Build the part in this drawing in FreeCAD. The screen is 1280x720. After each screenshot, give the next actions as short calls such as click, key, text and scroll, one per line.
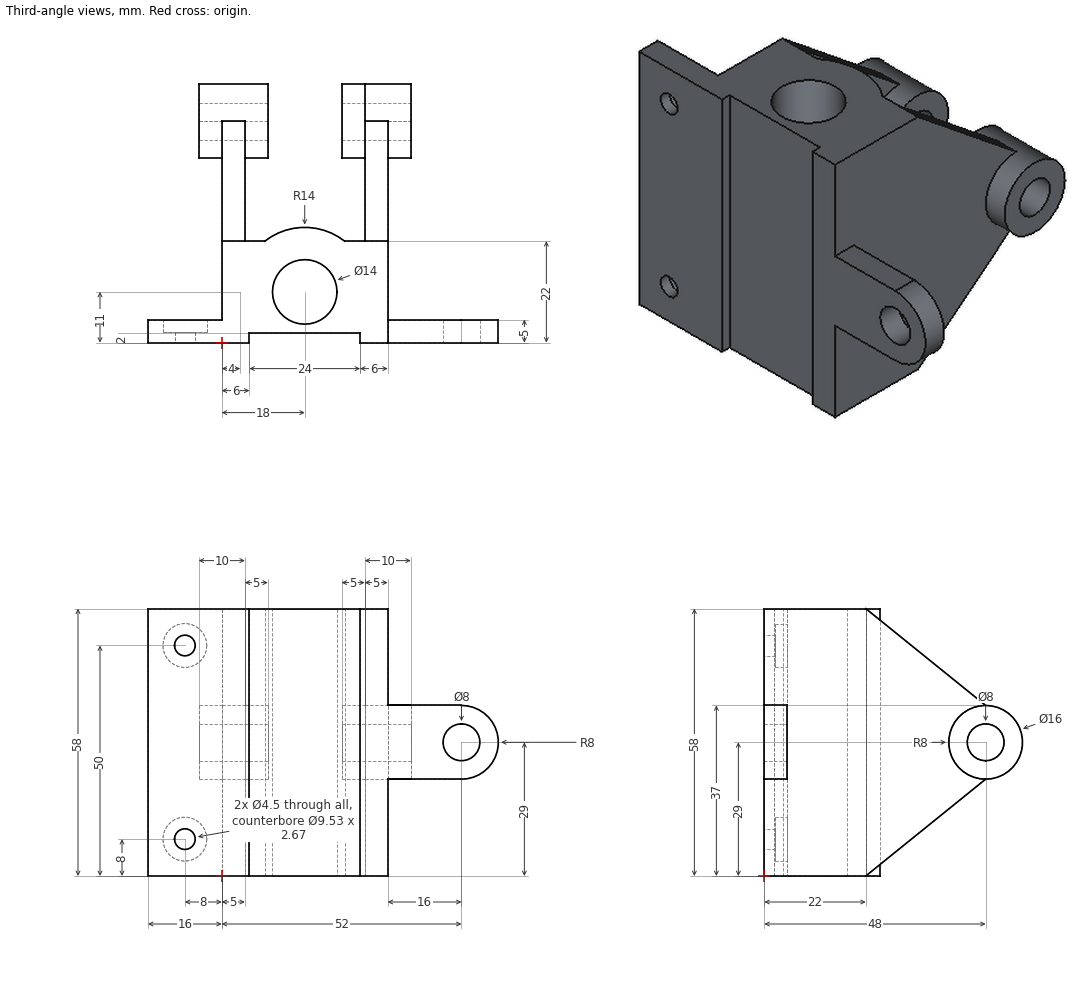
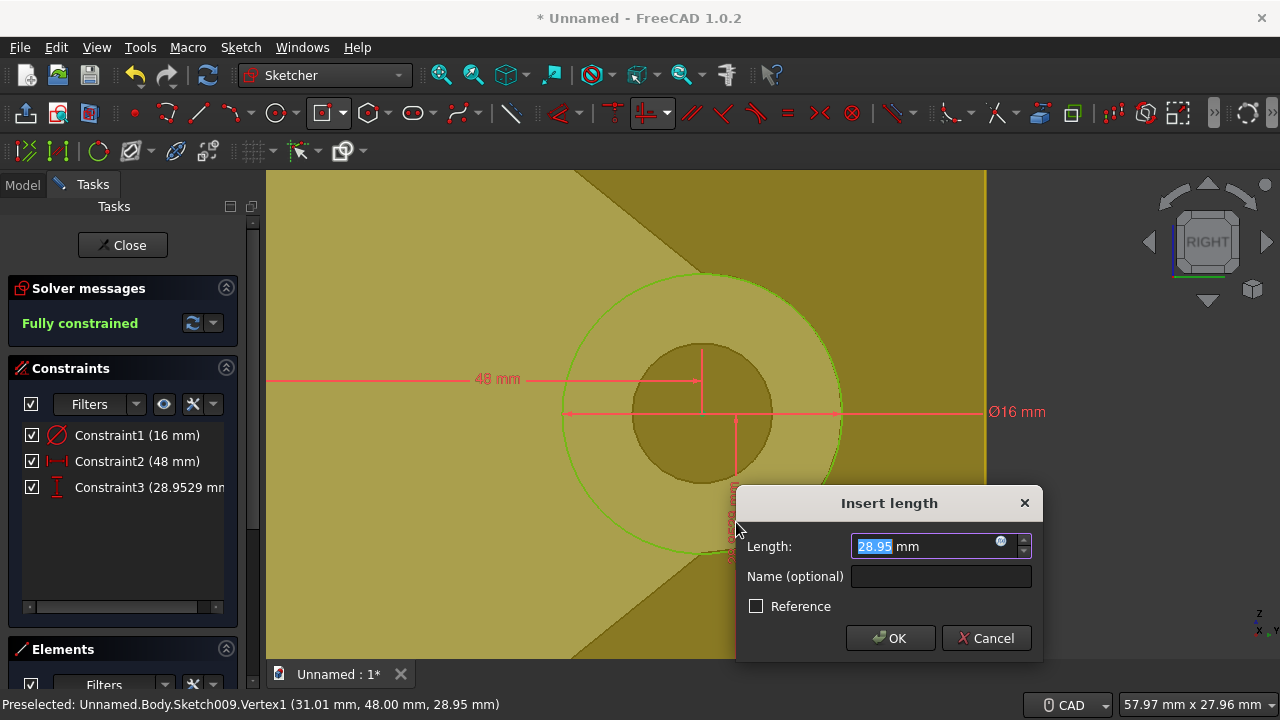
text(29)
key(Return)
key(Escape)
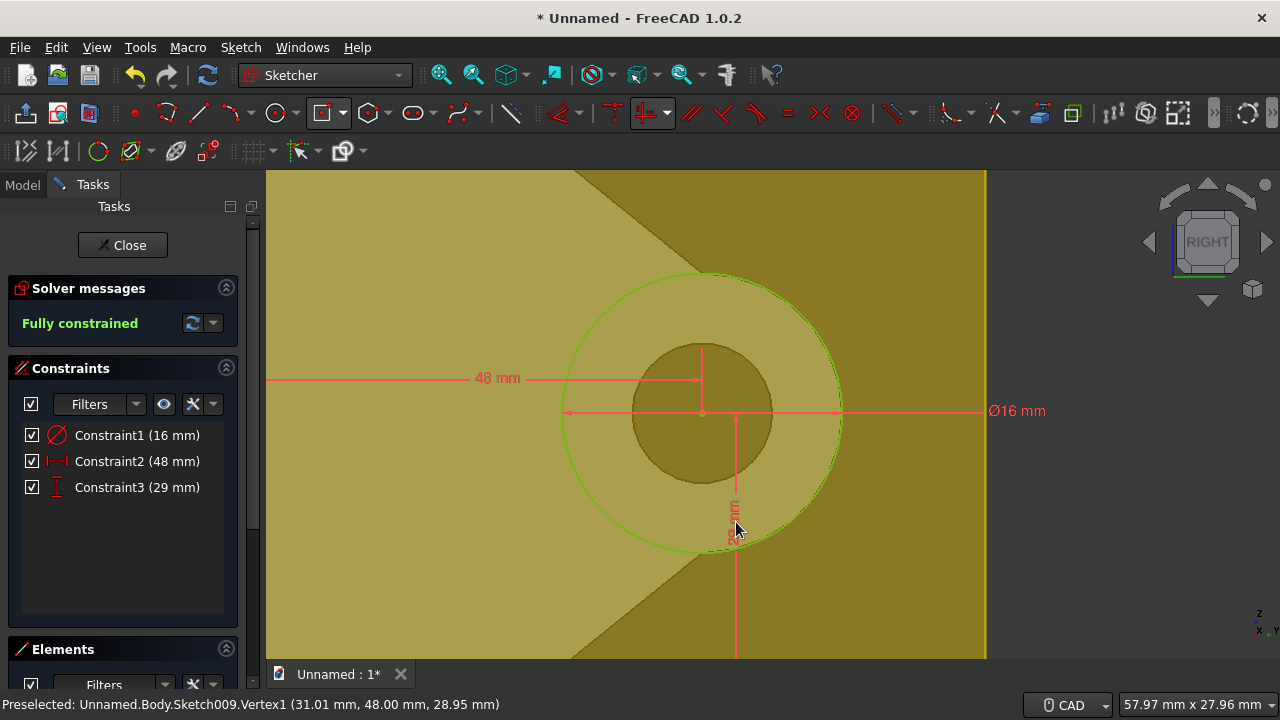
click(123, 245)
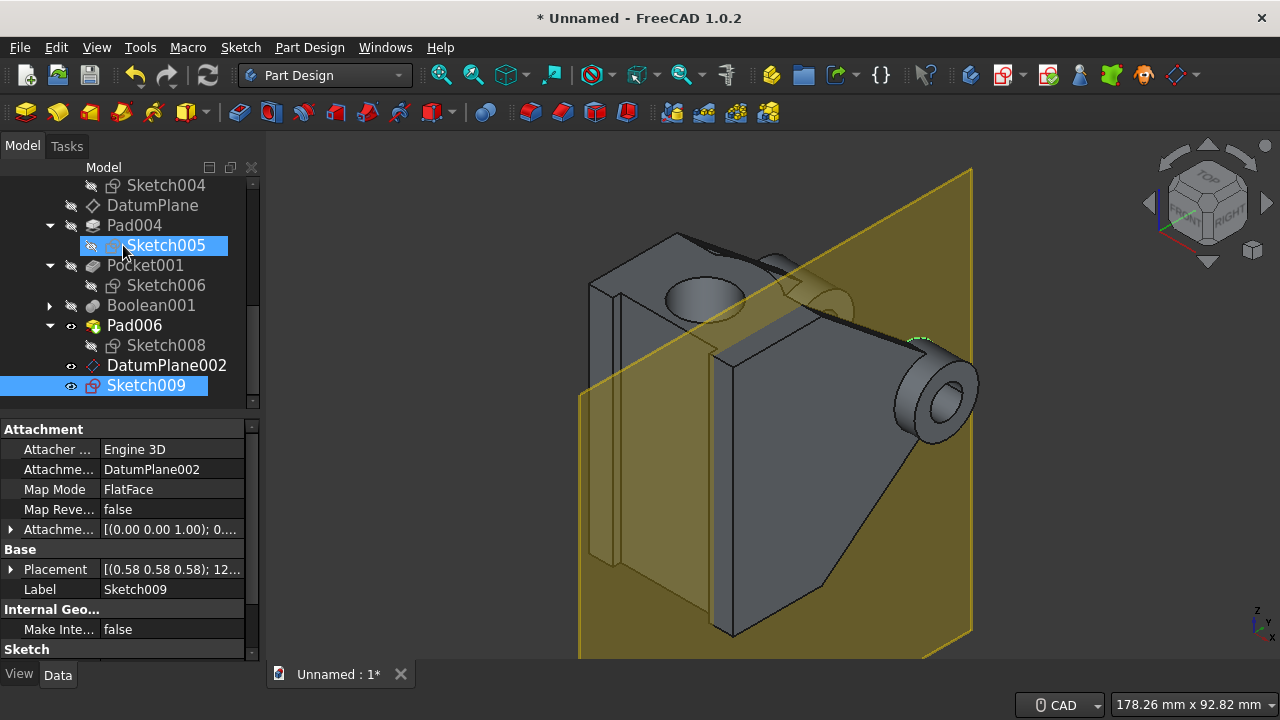
click(26, 112)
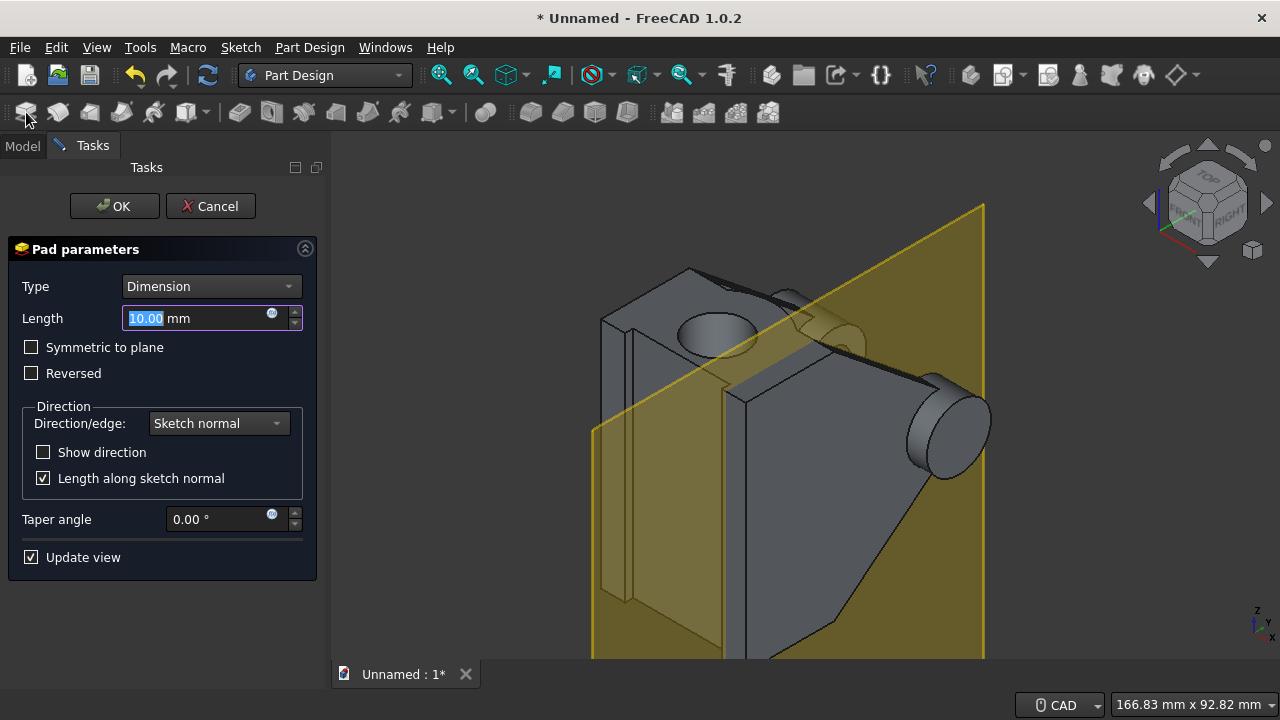
text(5)
key(Tab)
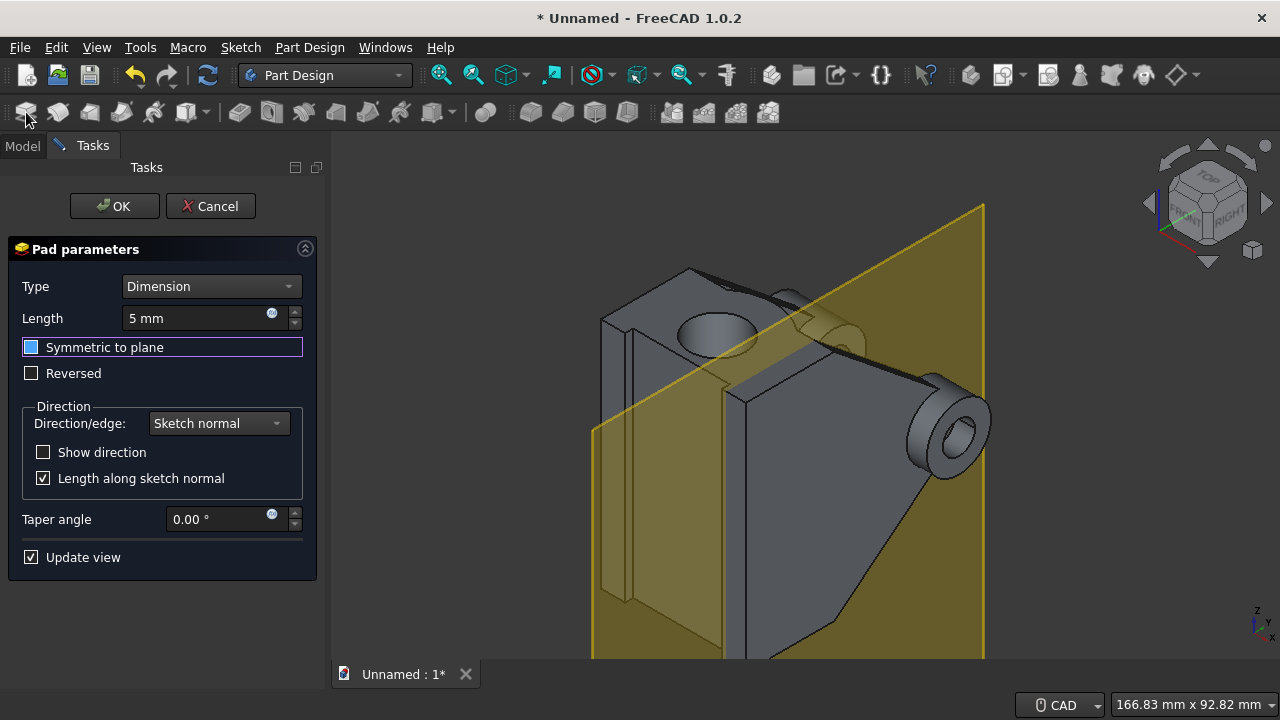
click(30, 373)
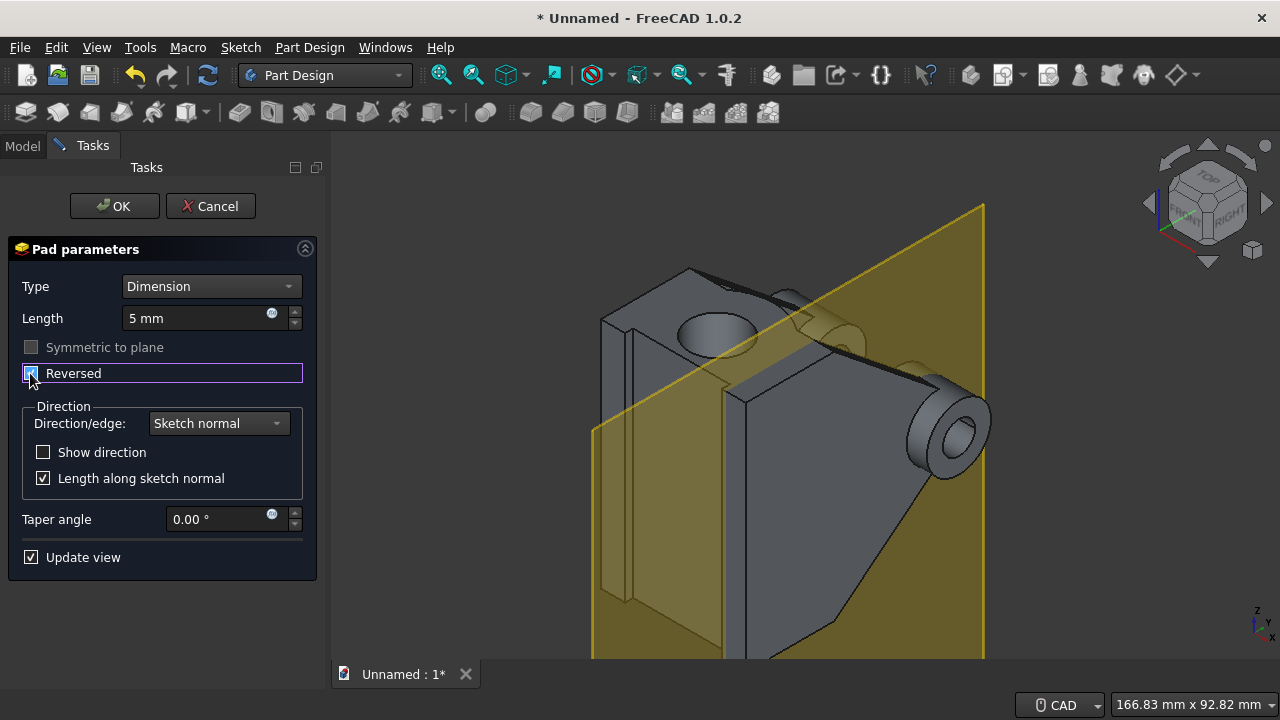
click(115, 206)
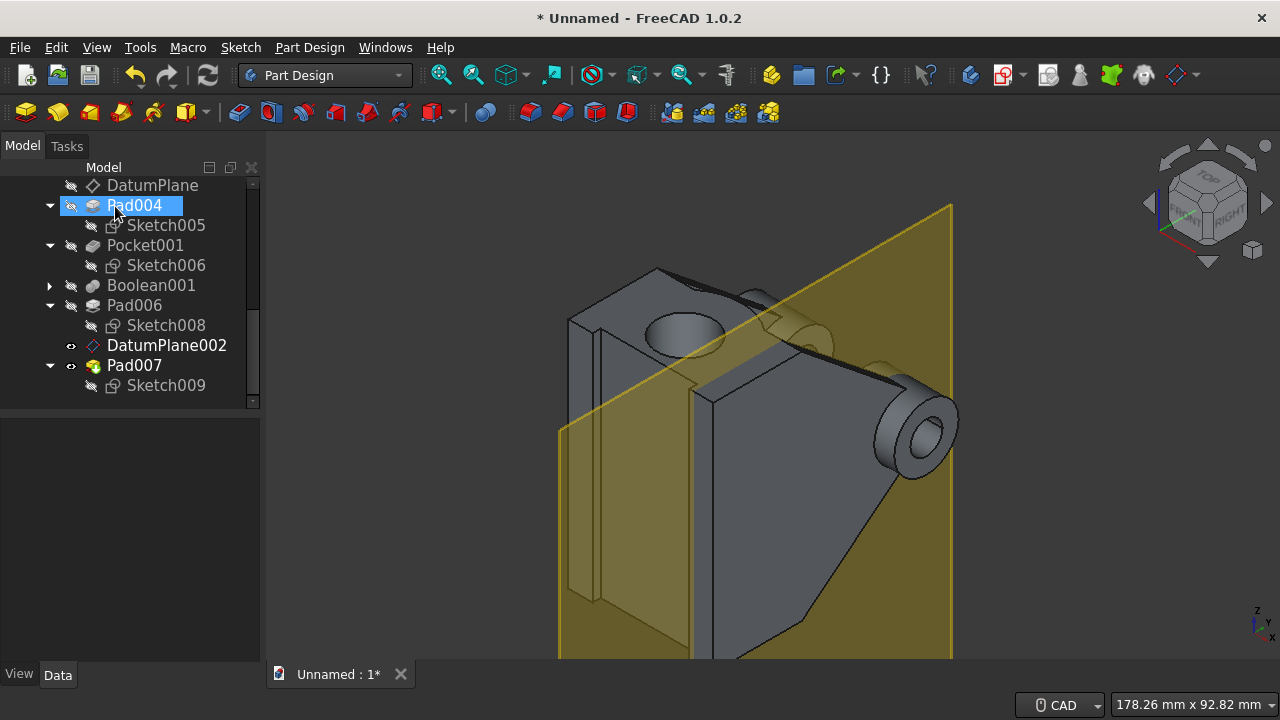
click(116, 346)
key(space)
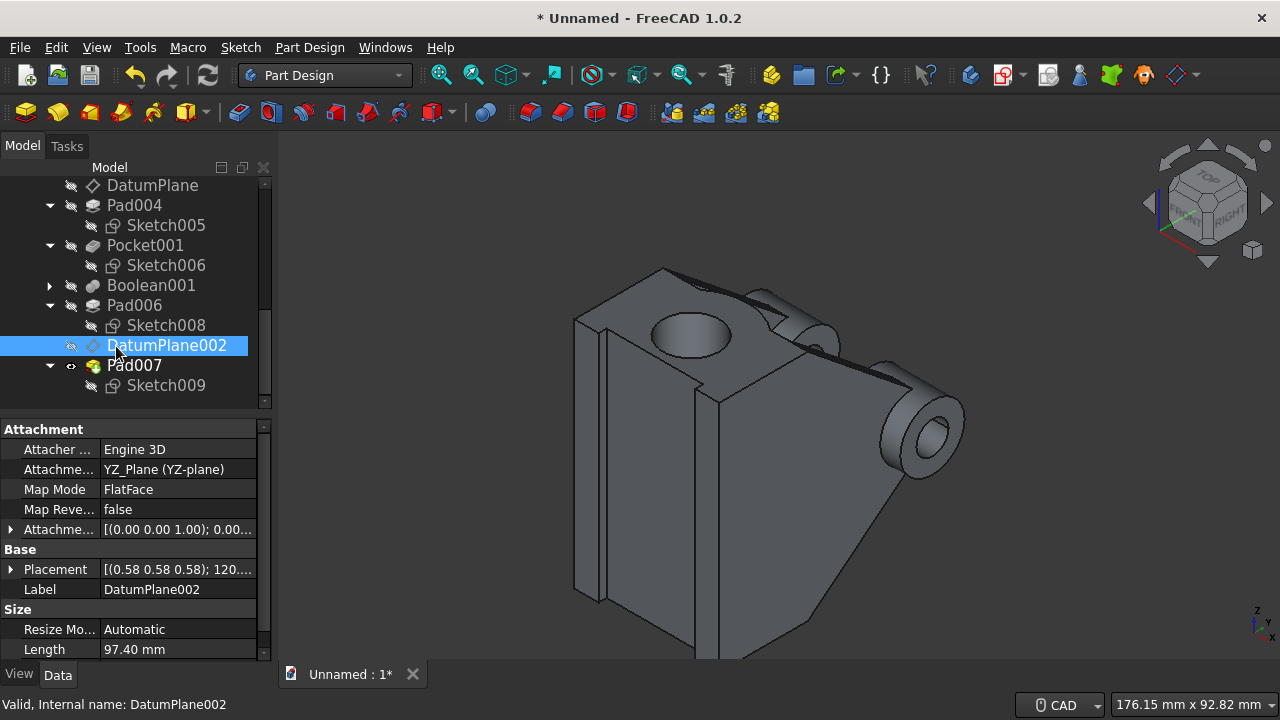
key(v)
key(f)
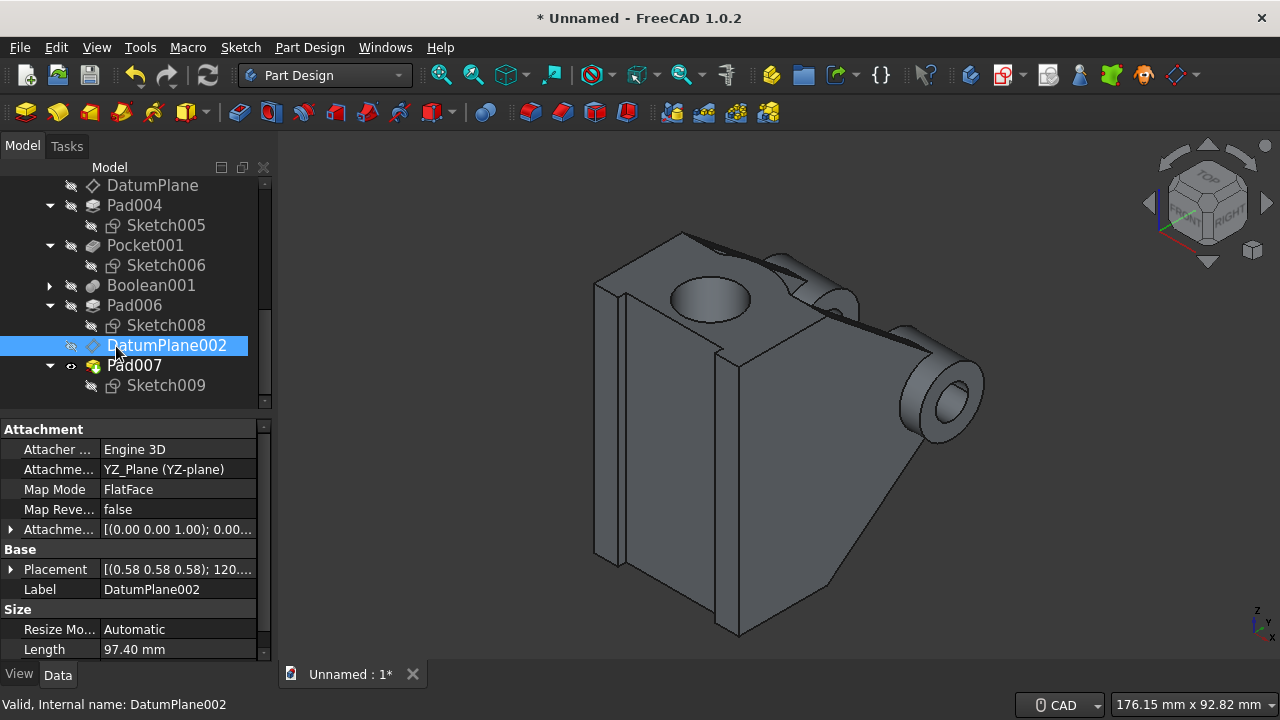
key(6)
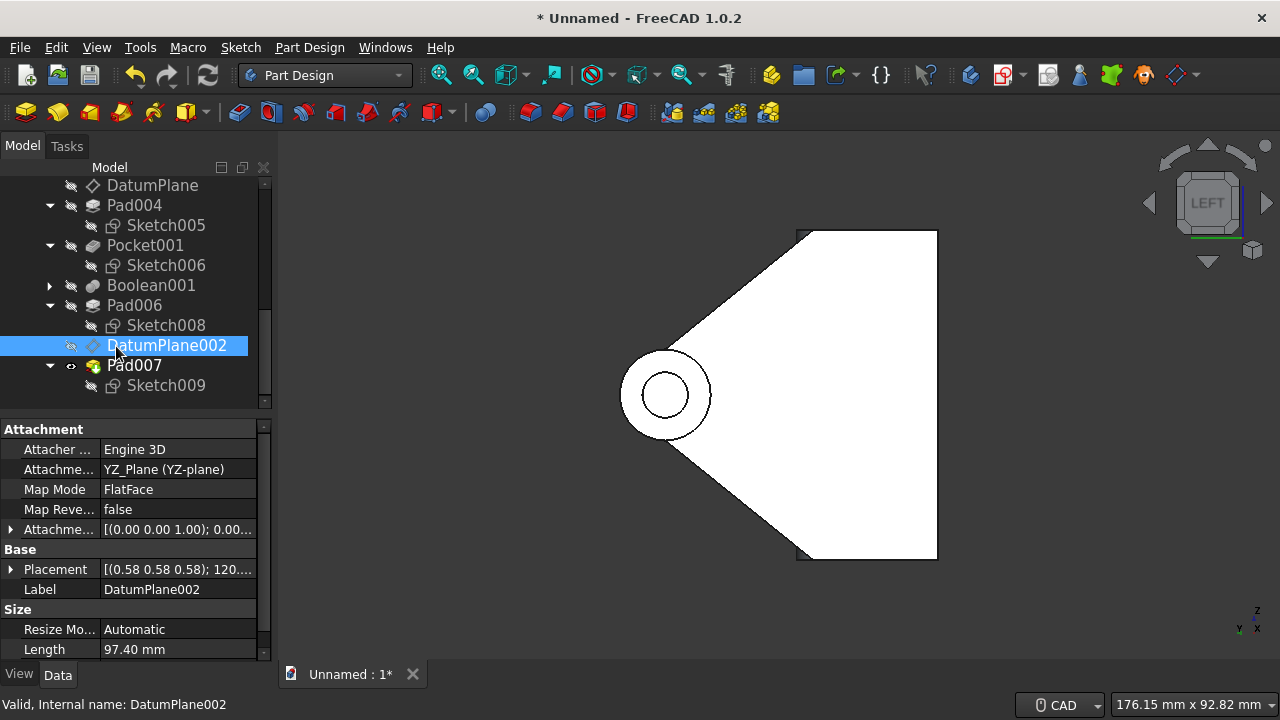
click(665, 394)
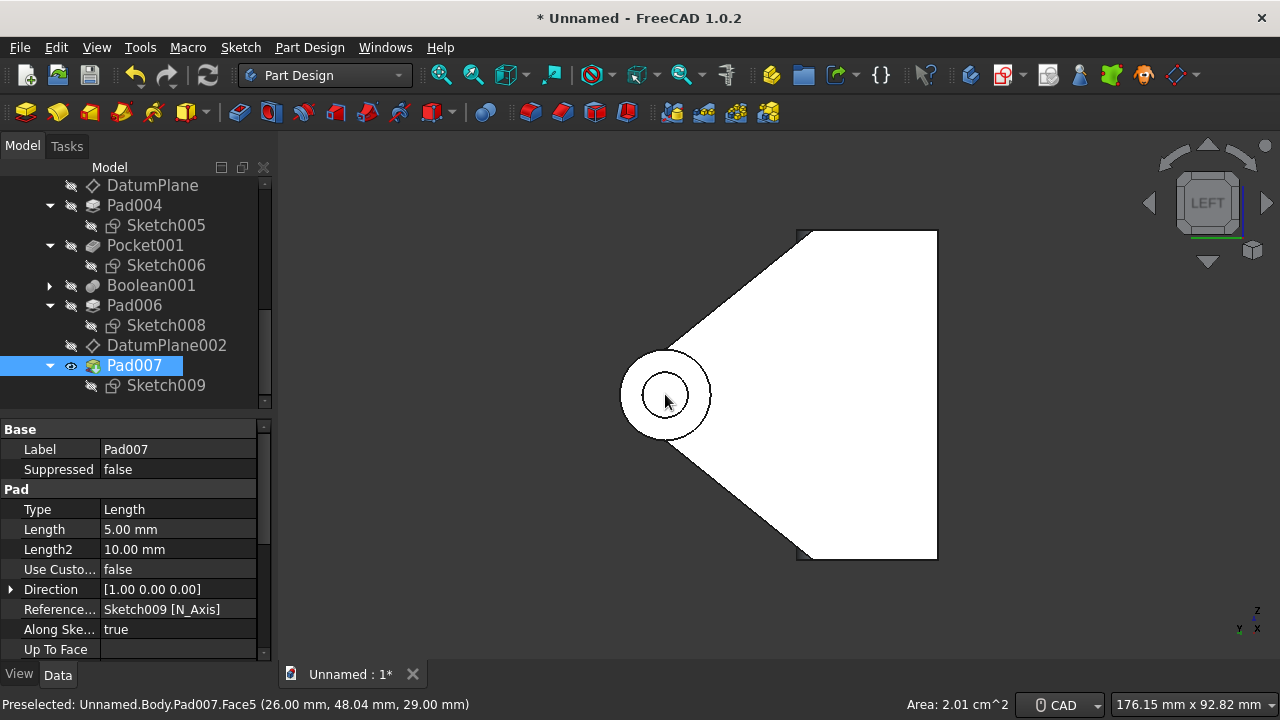
click(1004, 76)